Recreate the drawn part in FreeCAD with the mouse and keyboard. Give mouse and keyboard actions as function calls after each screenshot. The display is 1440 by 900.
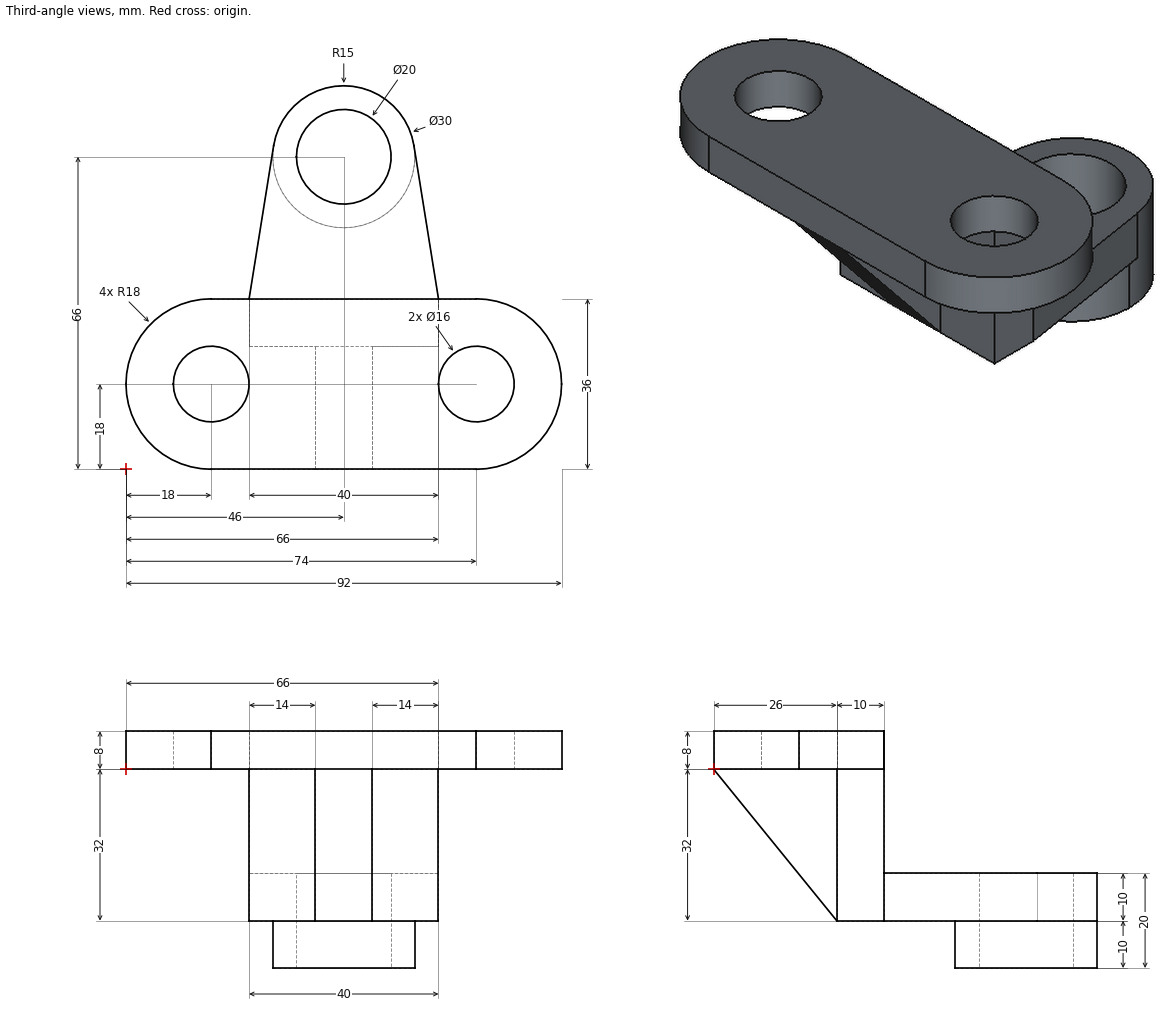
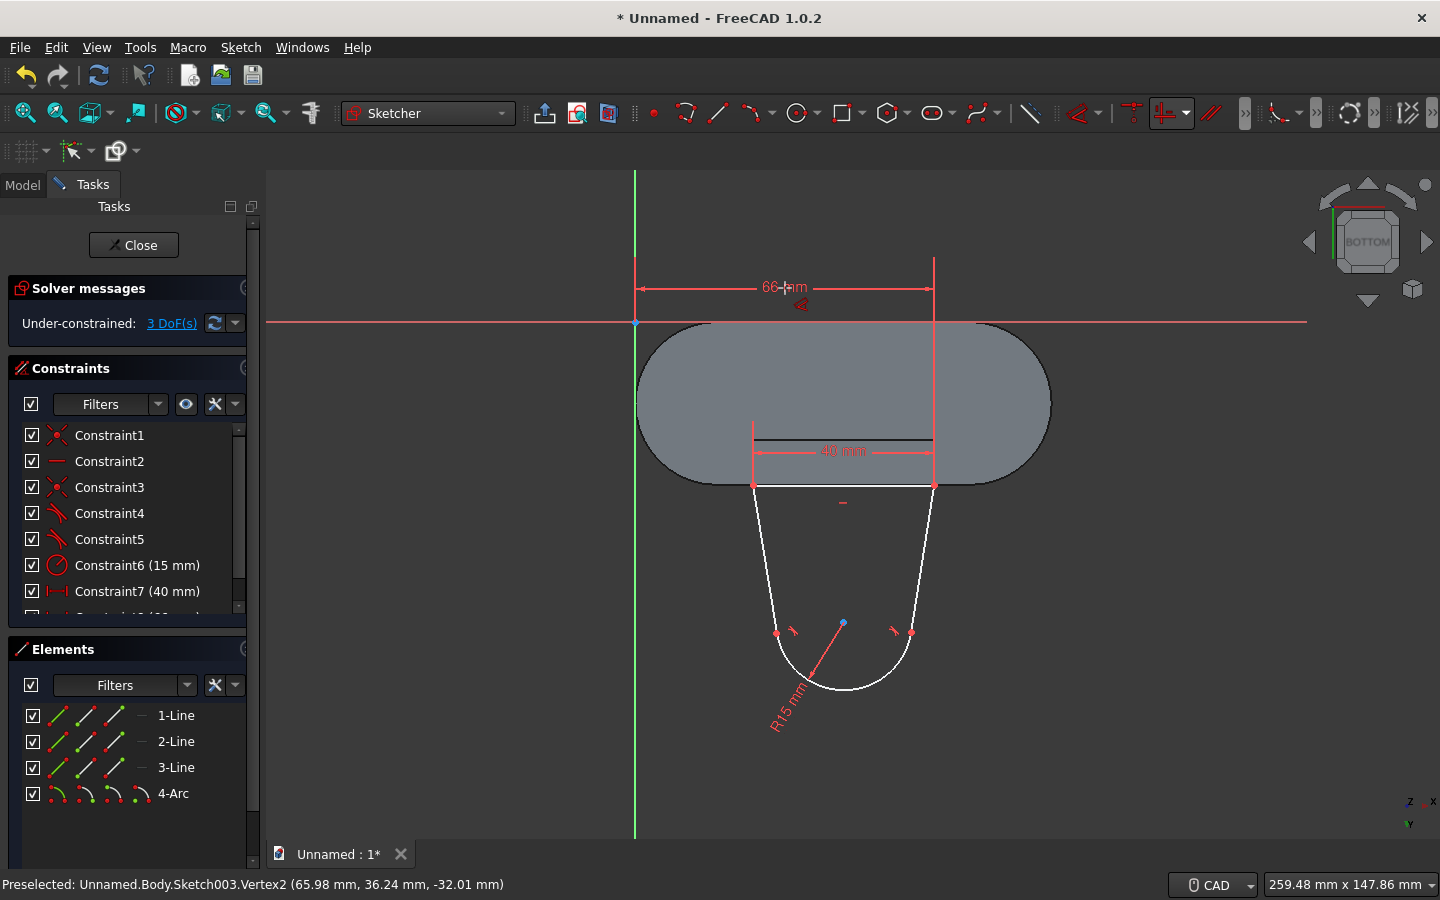
click(934, 486)
click(968, 404)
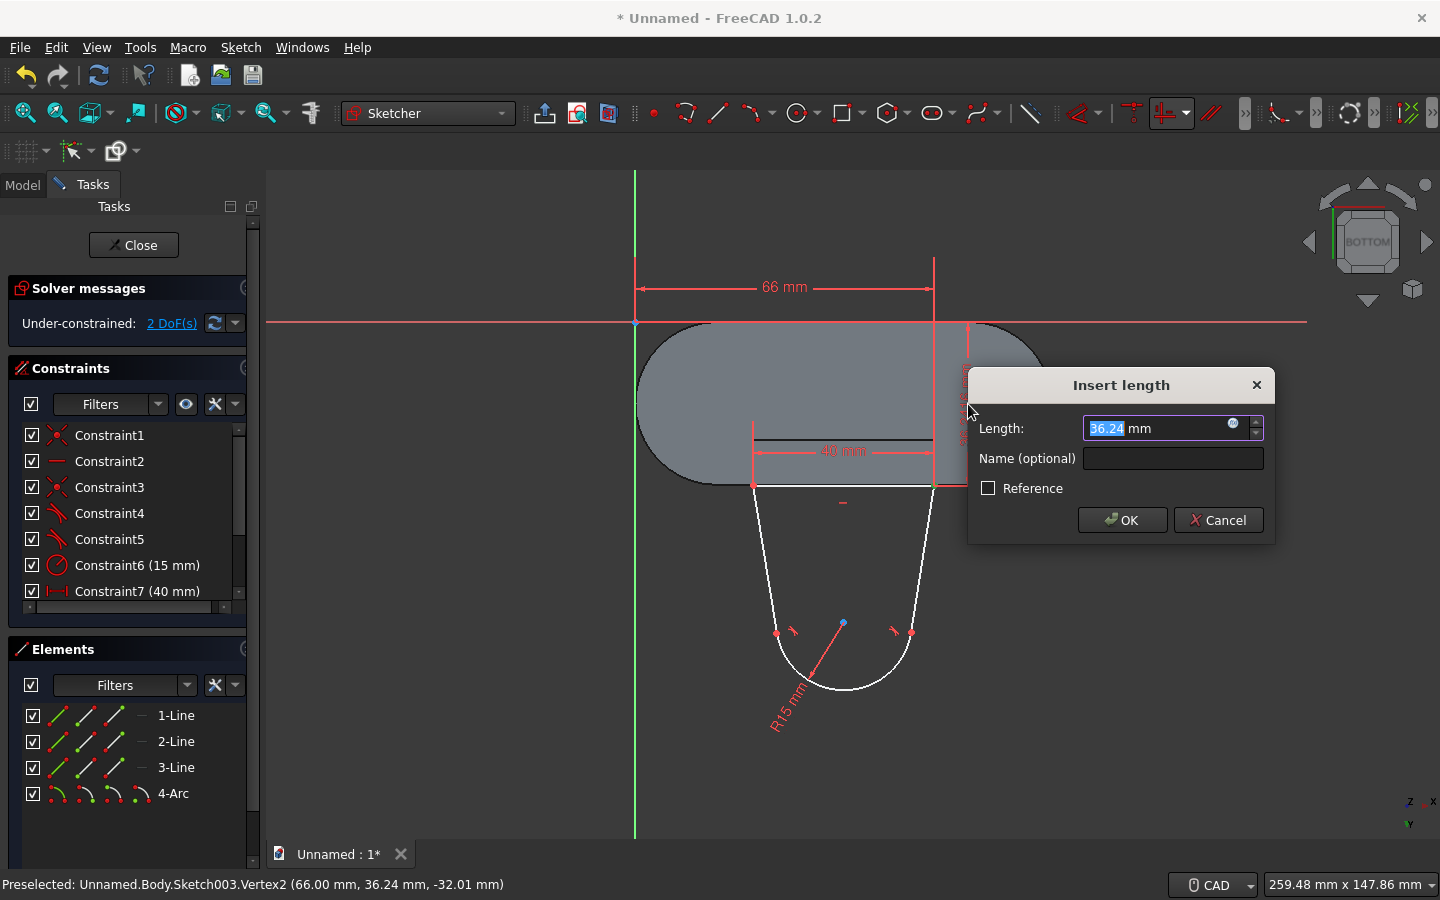
text(36)
key(Return)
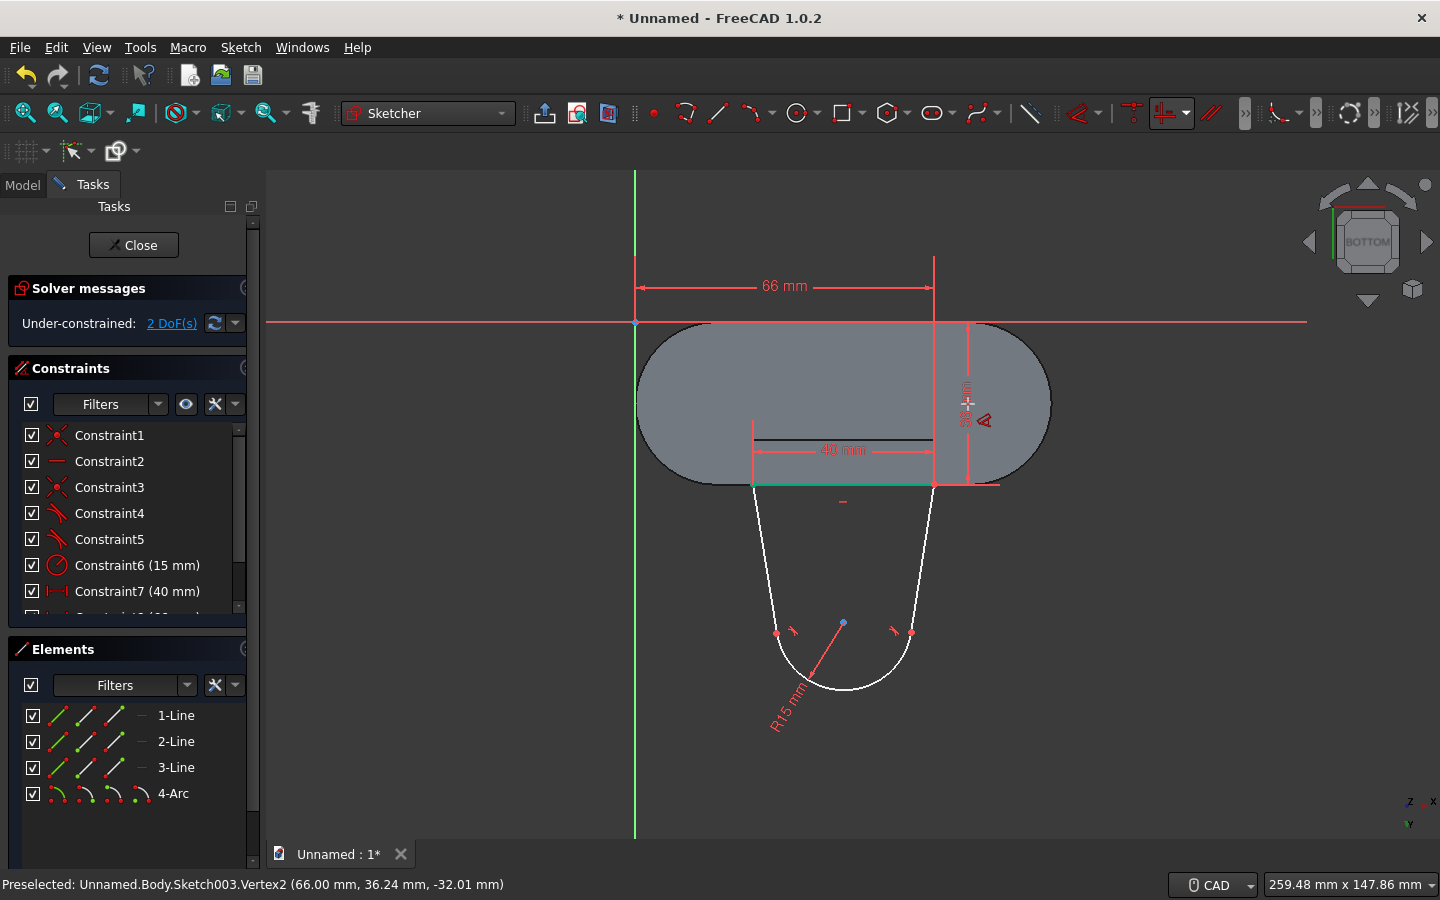
click(844, 622)
click(692, 288)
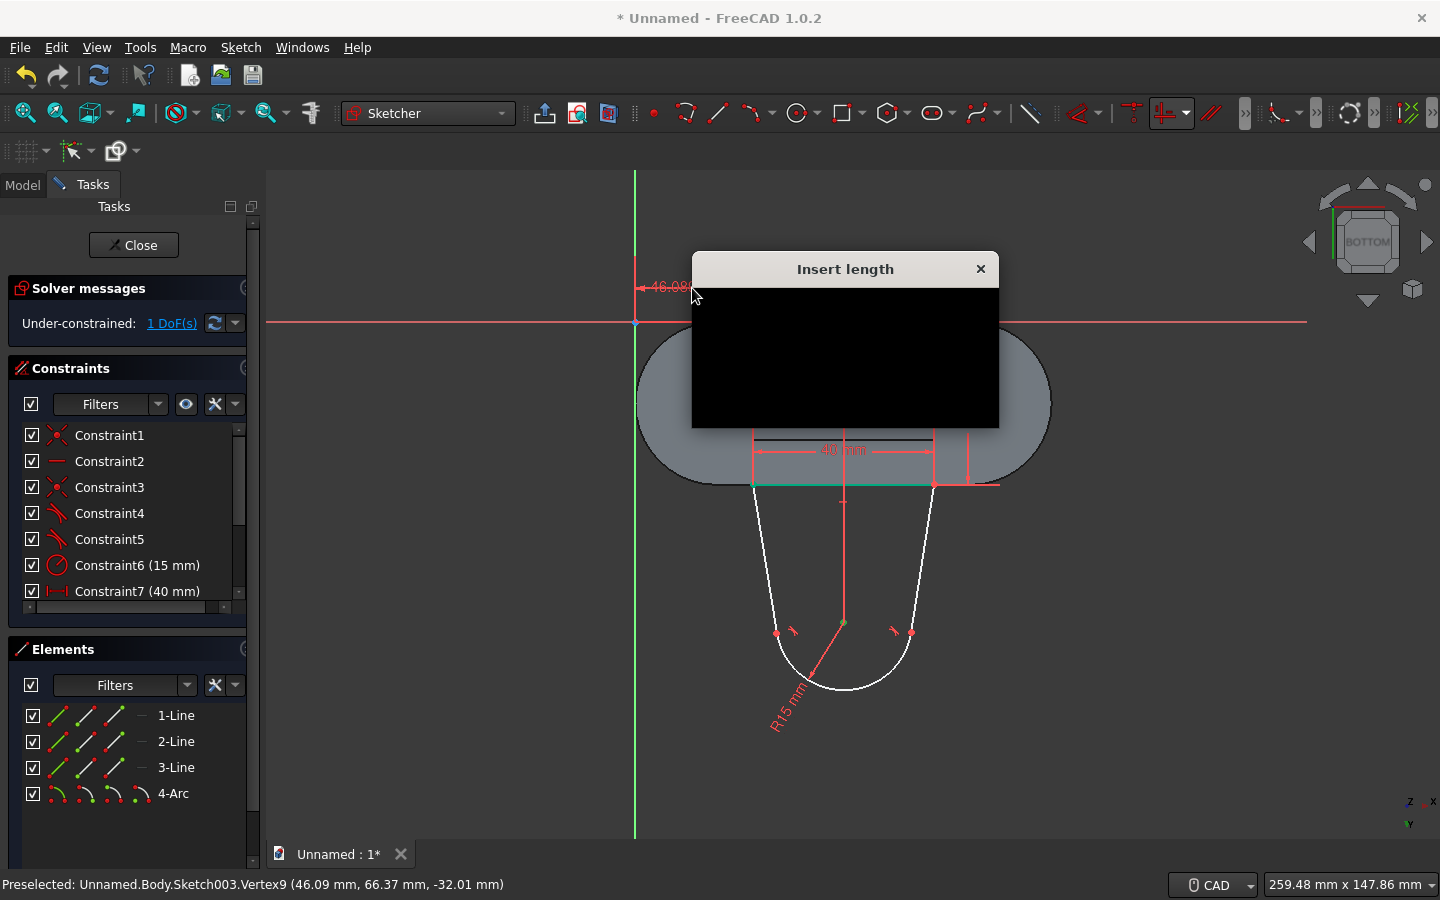
text(46)
key(Return)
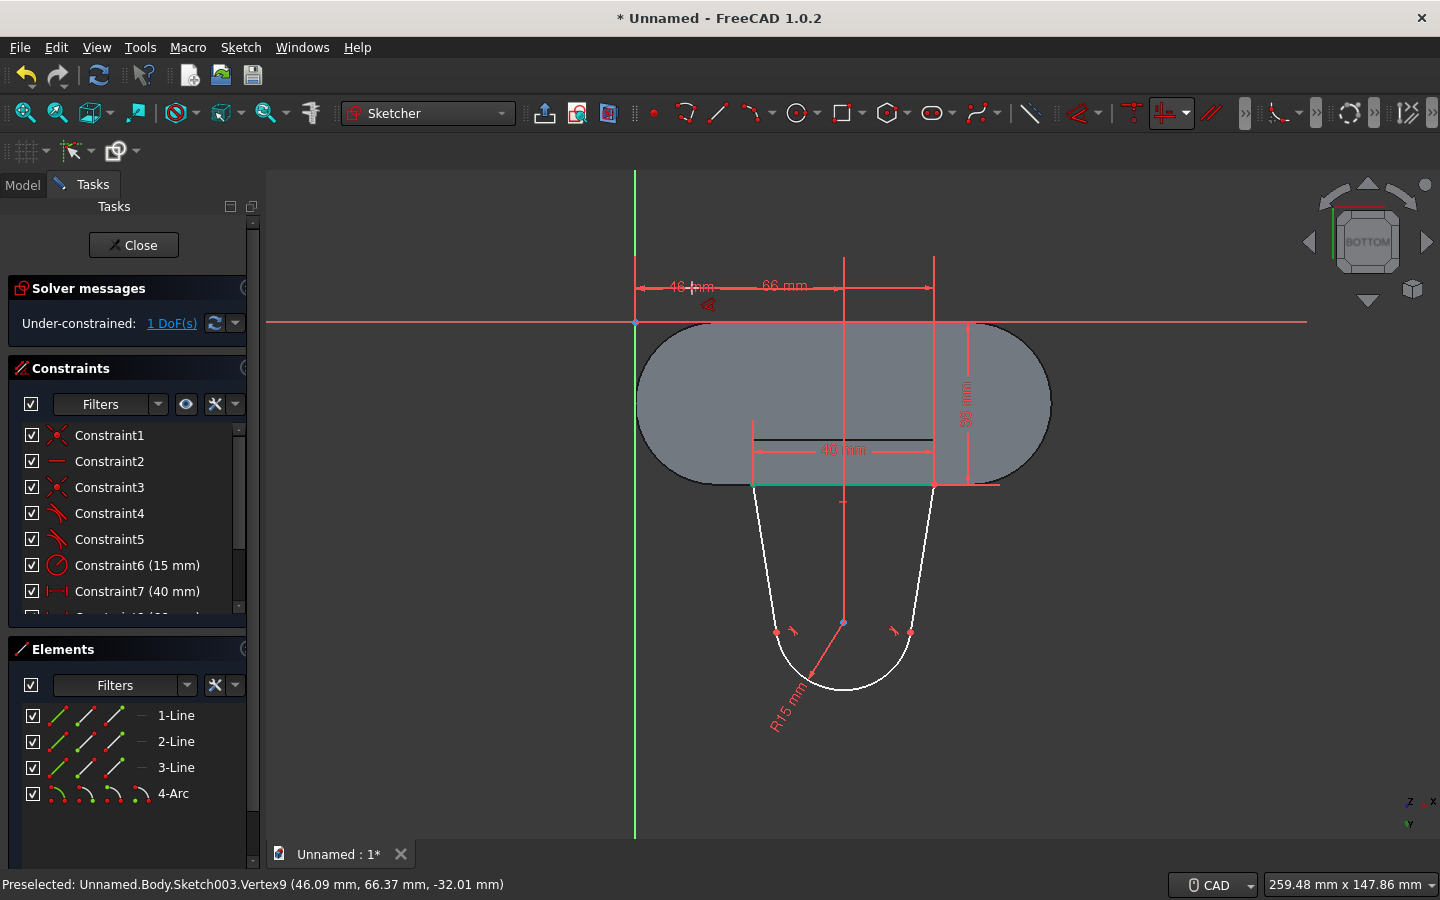
click(844, 622)
click(601, 472)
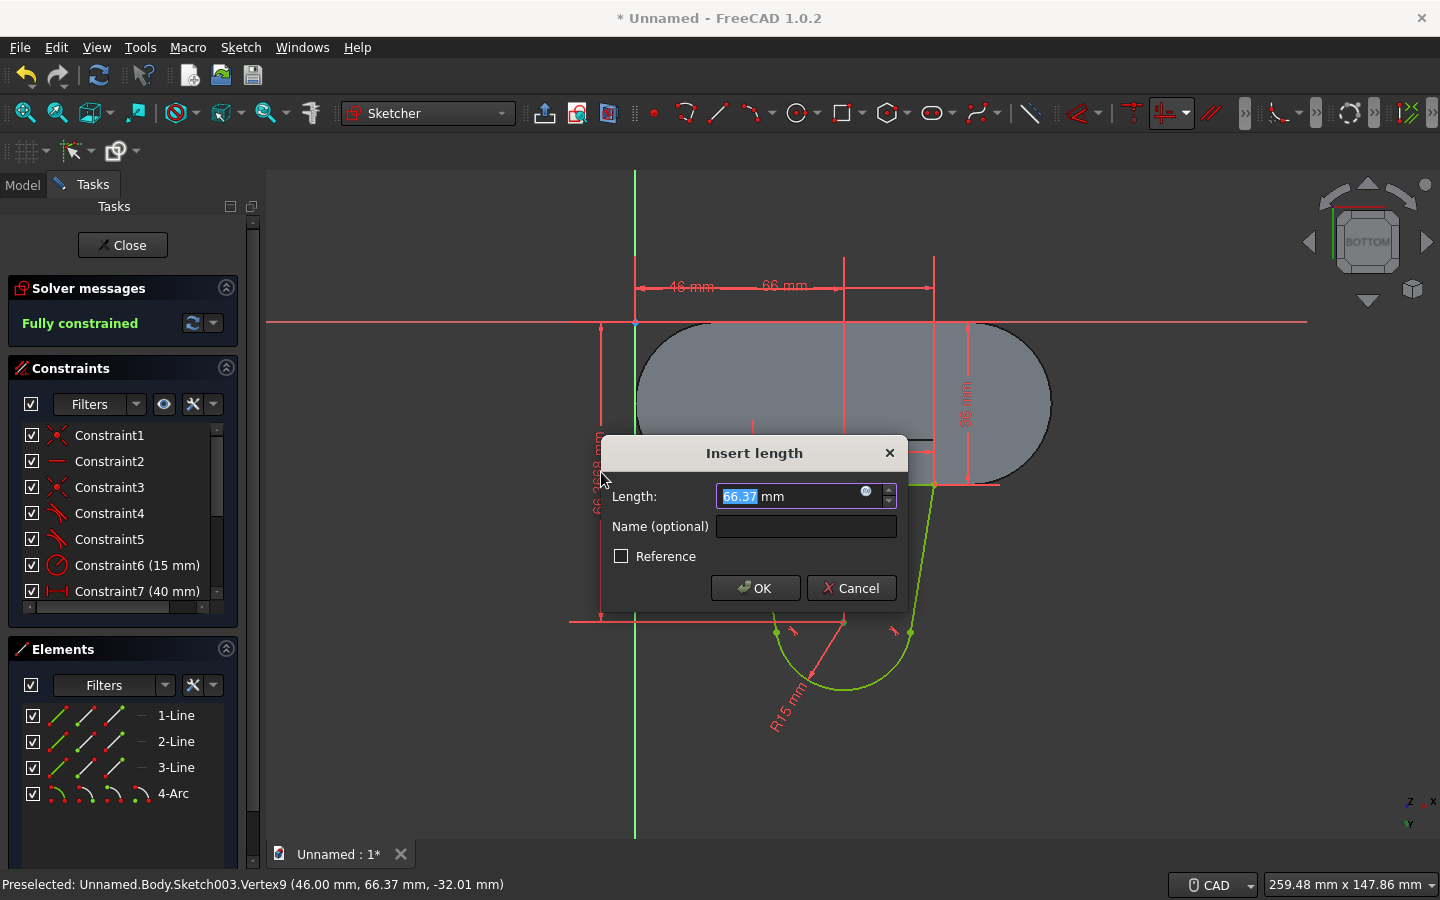
text(66)
key(Return)
key(Escape)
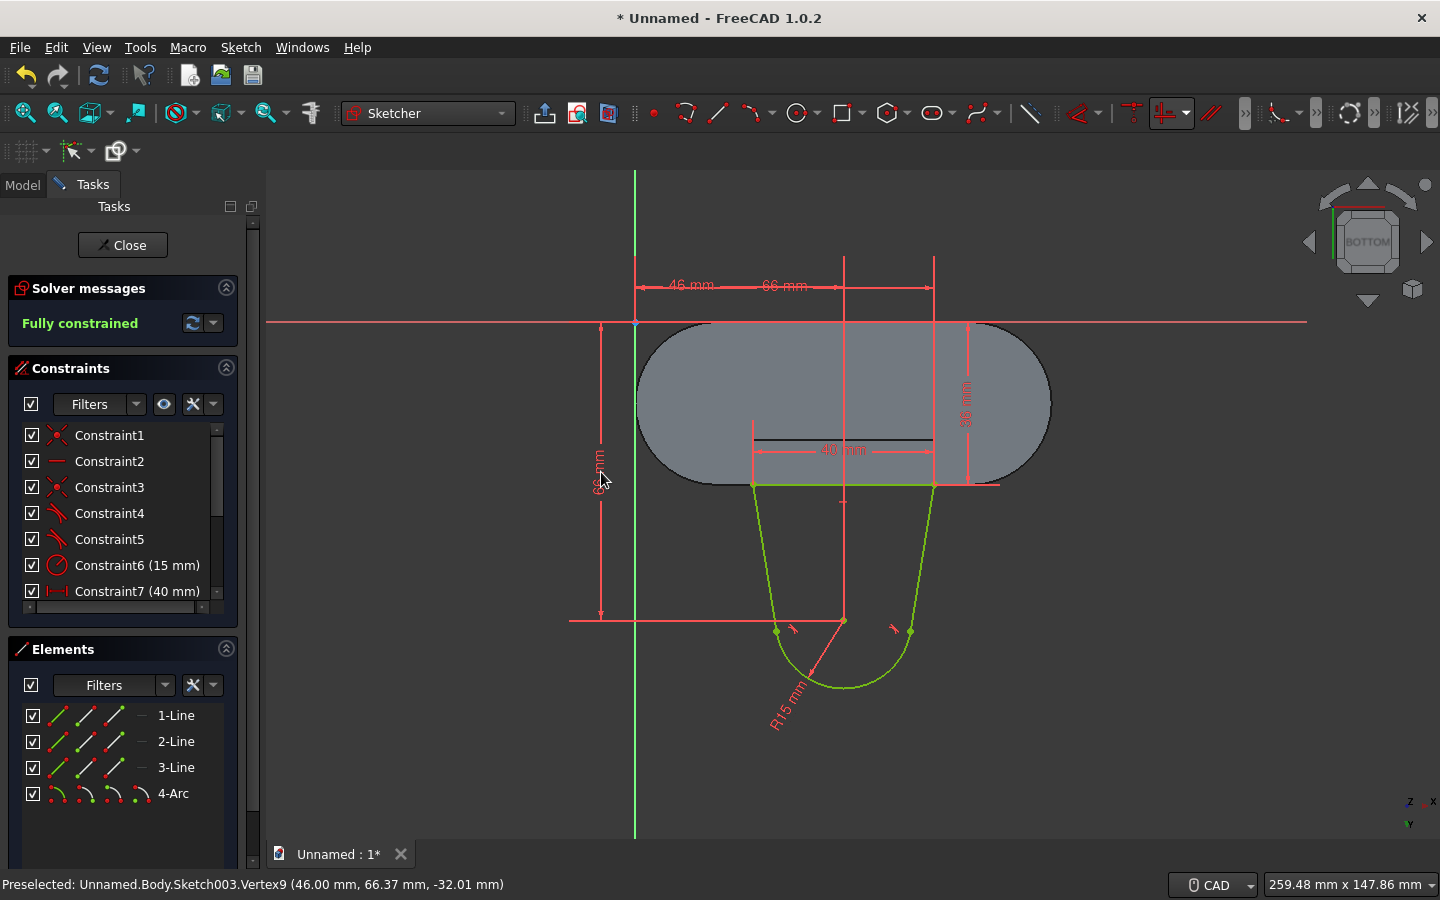
click(123, 245)